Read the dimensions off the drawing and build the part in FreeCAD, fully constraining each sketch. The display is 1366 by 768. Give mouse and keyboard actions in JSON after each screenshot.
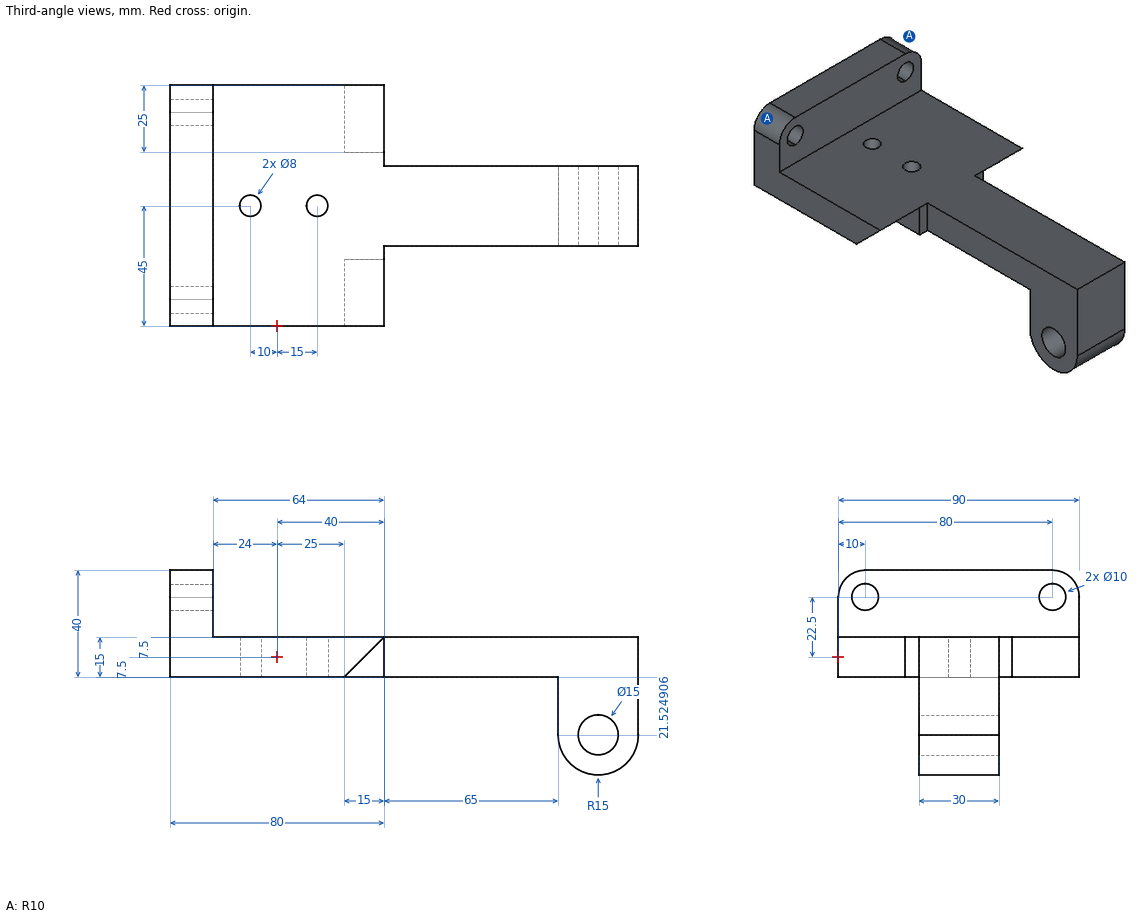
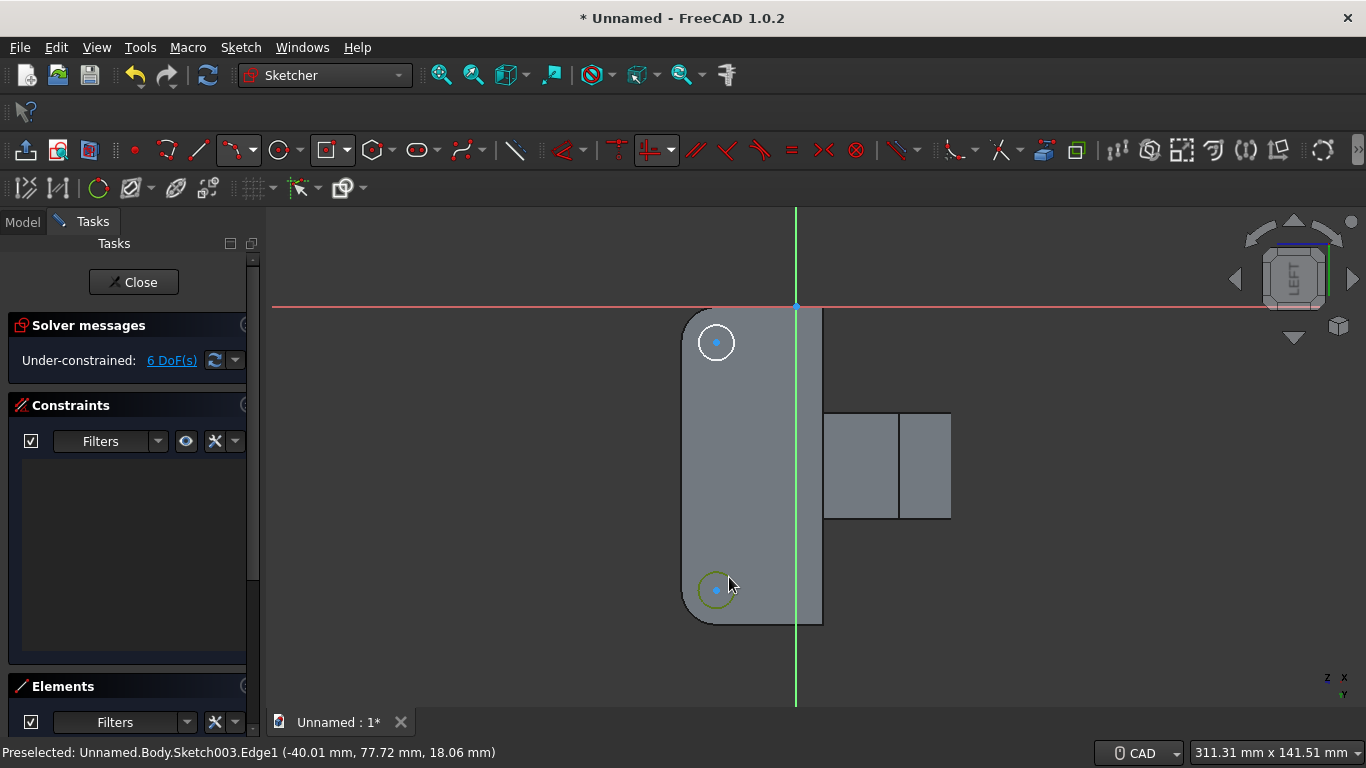
{"action": "left_click", "coordinate": [729, 330]}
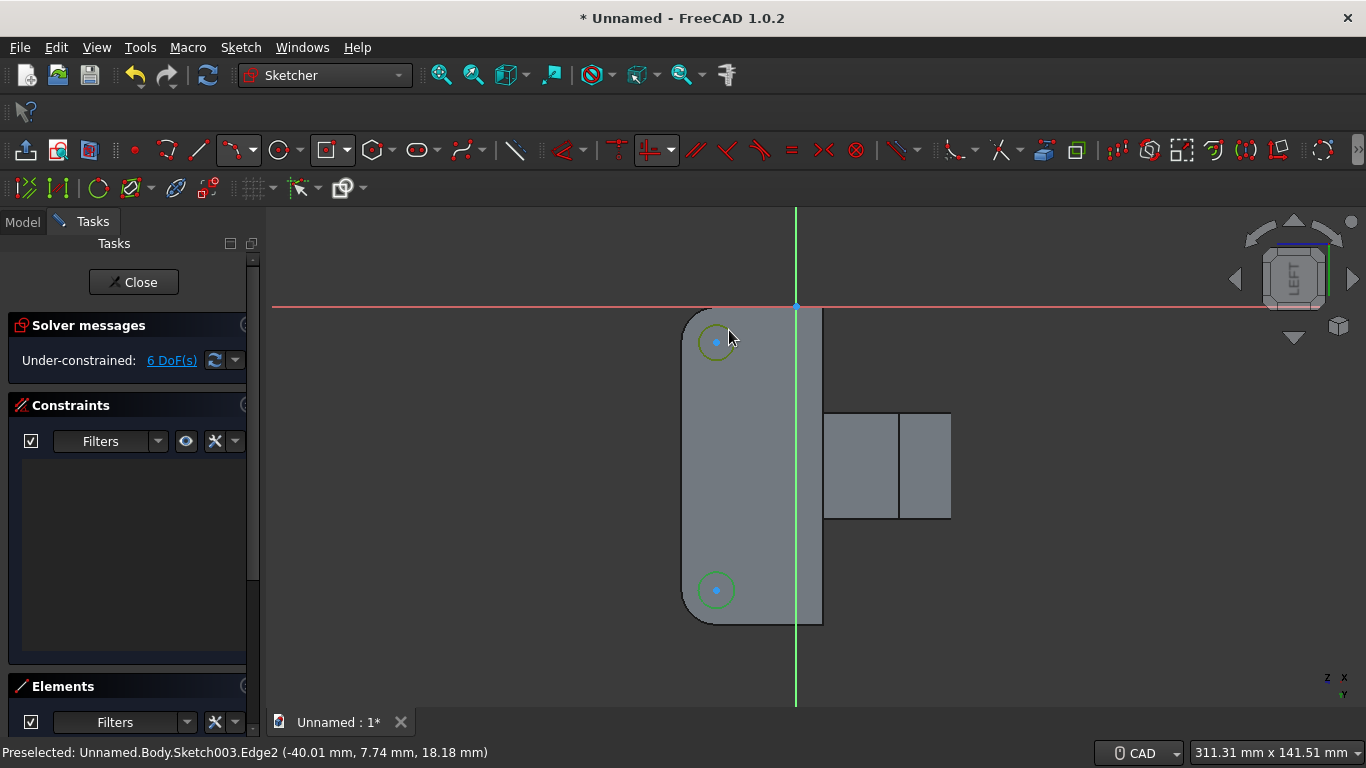
{"action": "left_click", "coordinate": [792, 150]}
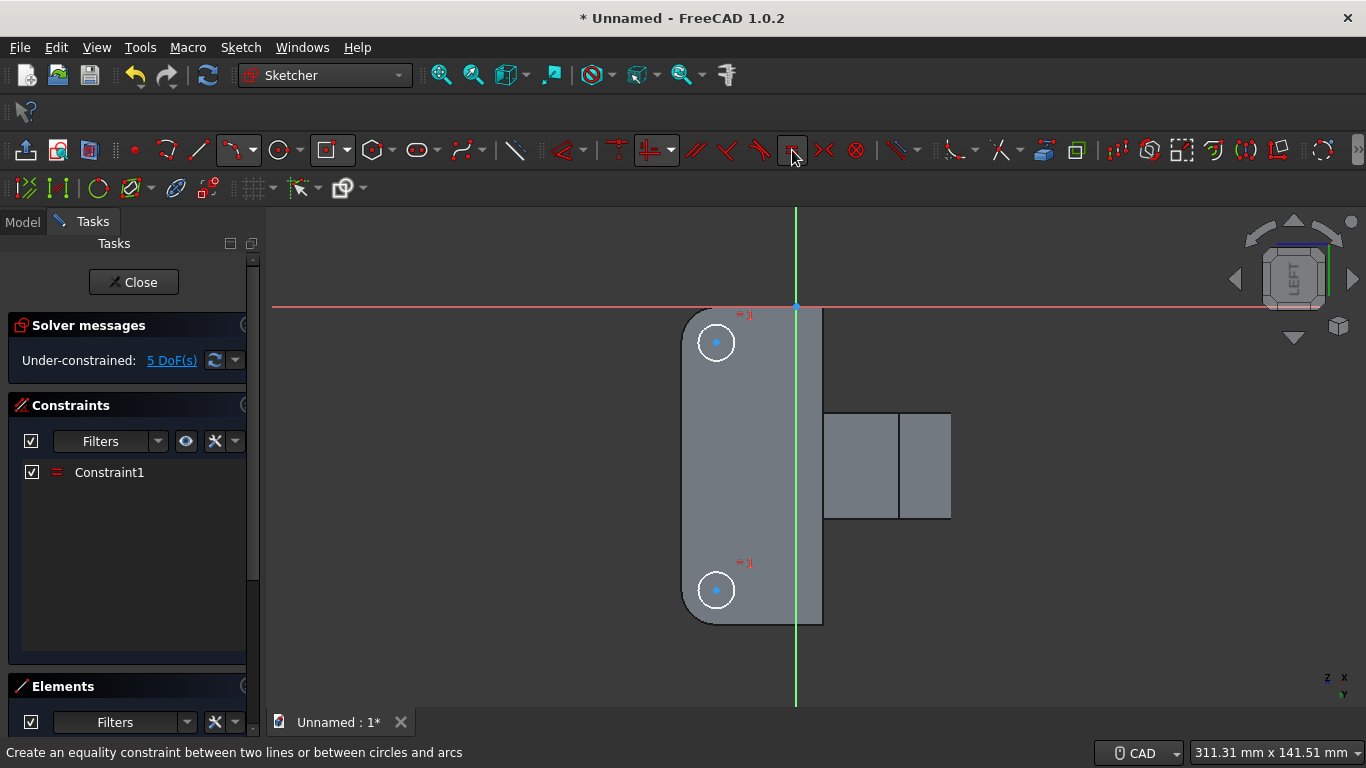
{"action": "left_click", "coordinate": [716, 590]}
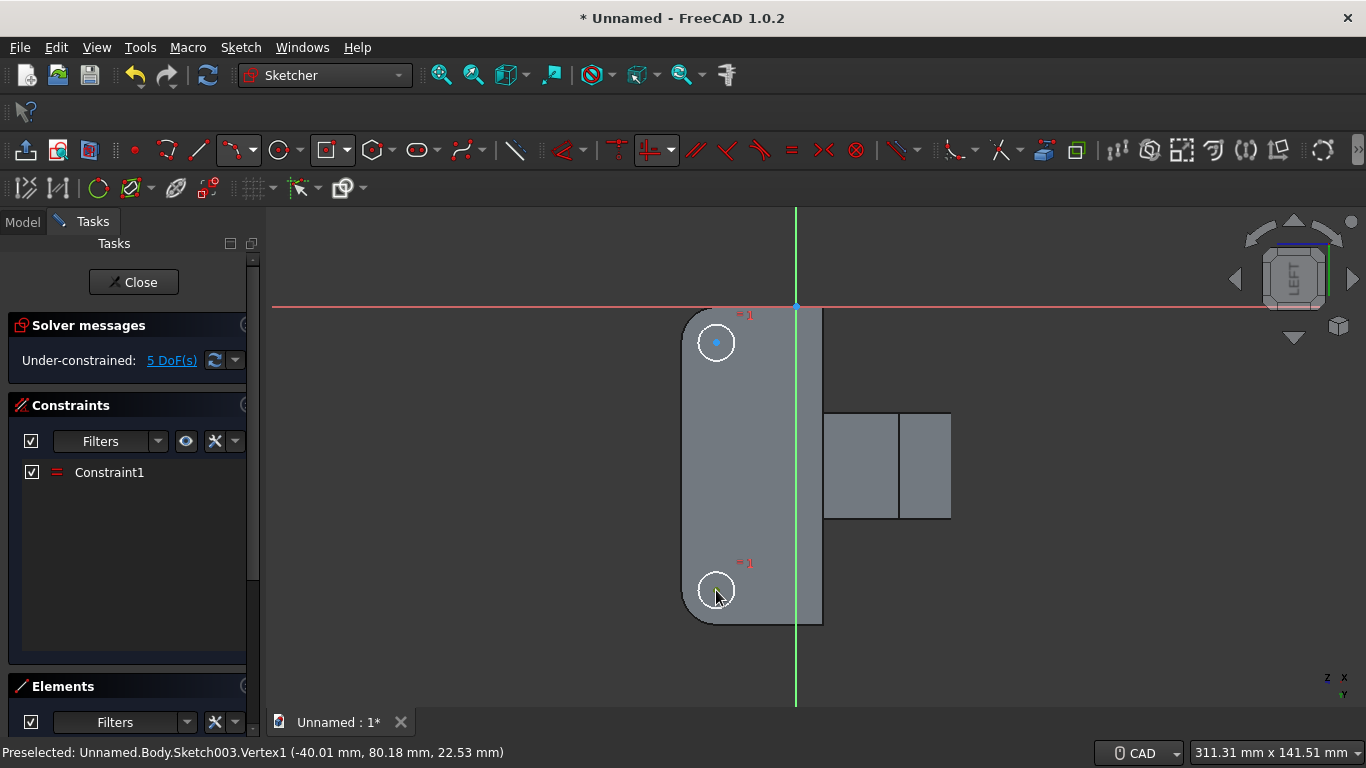
{"action": "left_click", "coordinate": [716, 343]}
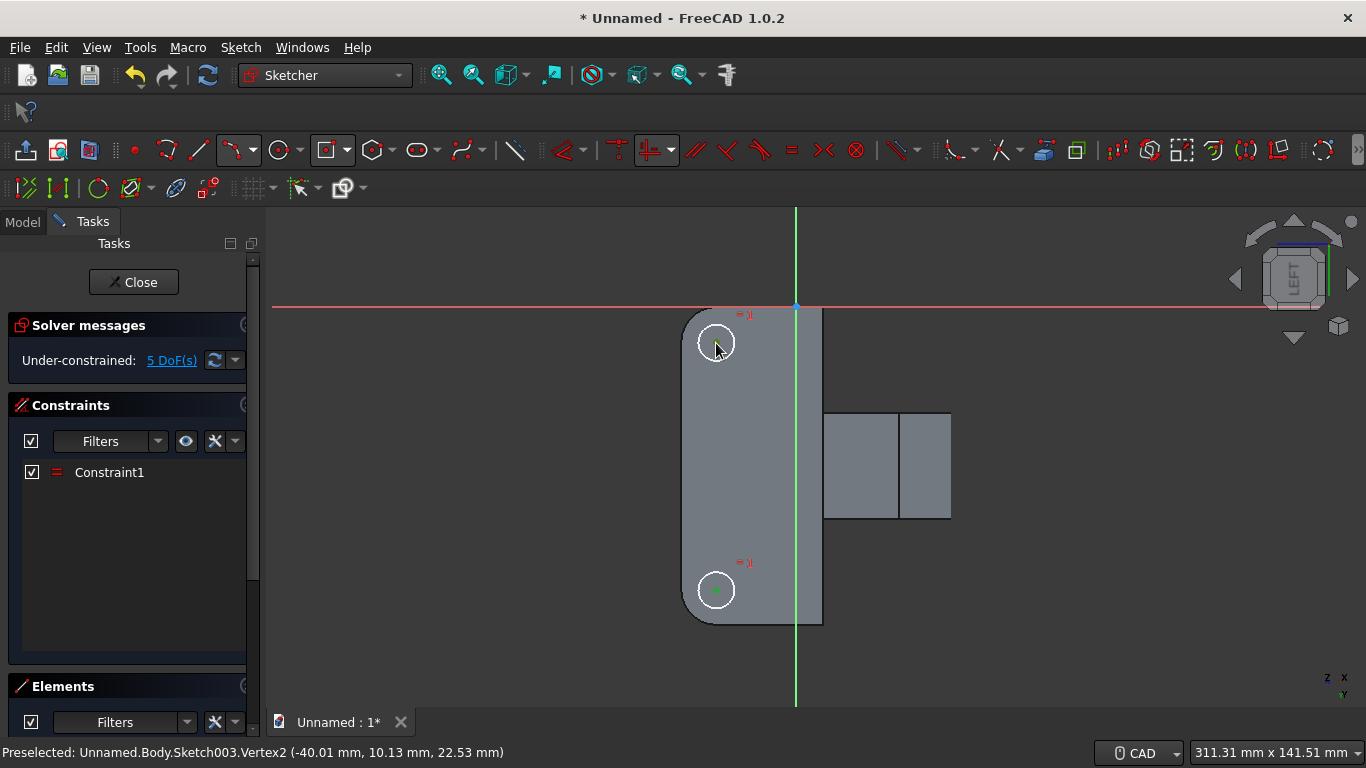
{"action": "left_click", "coordinate": [674, 150]}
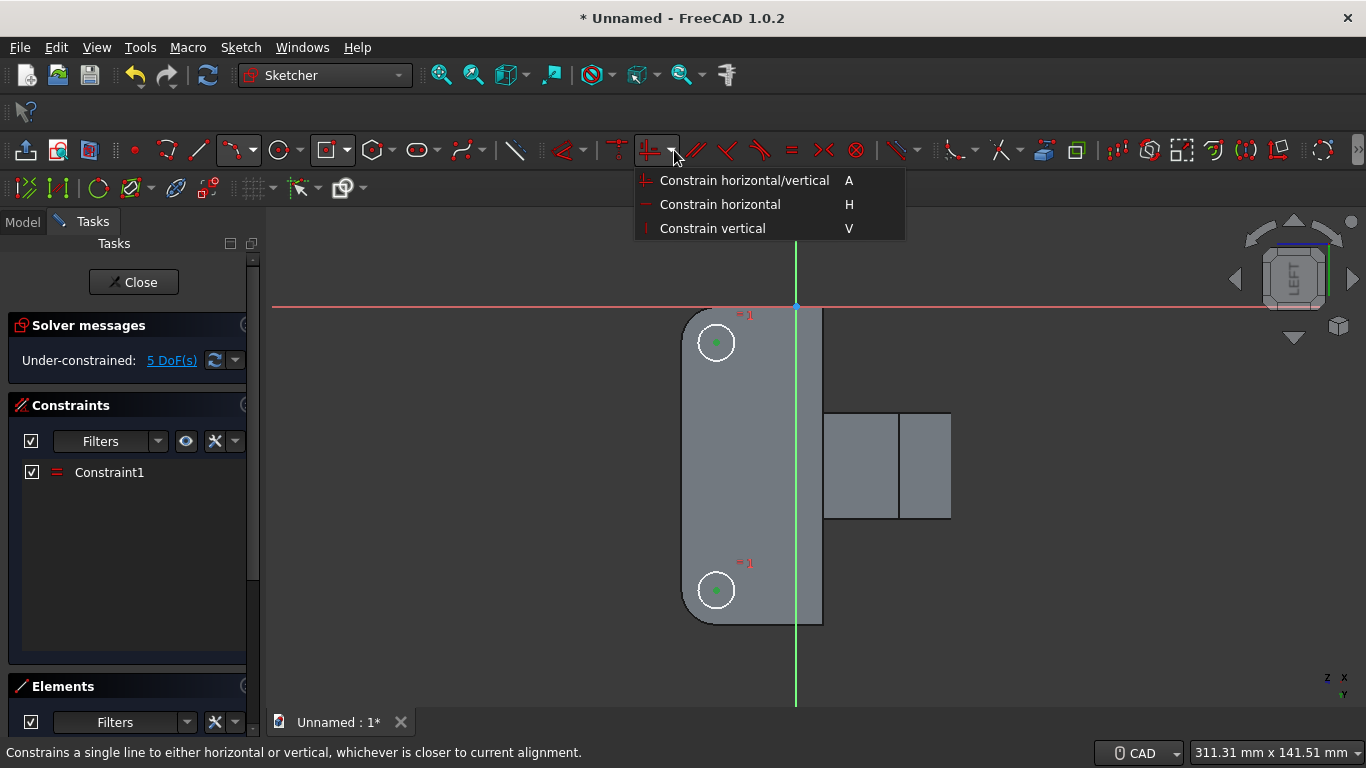
{"action": "left_click", "coordinate": [770, 228]}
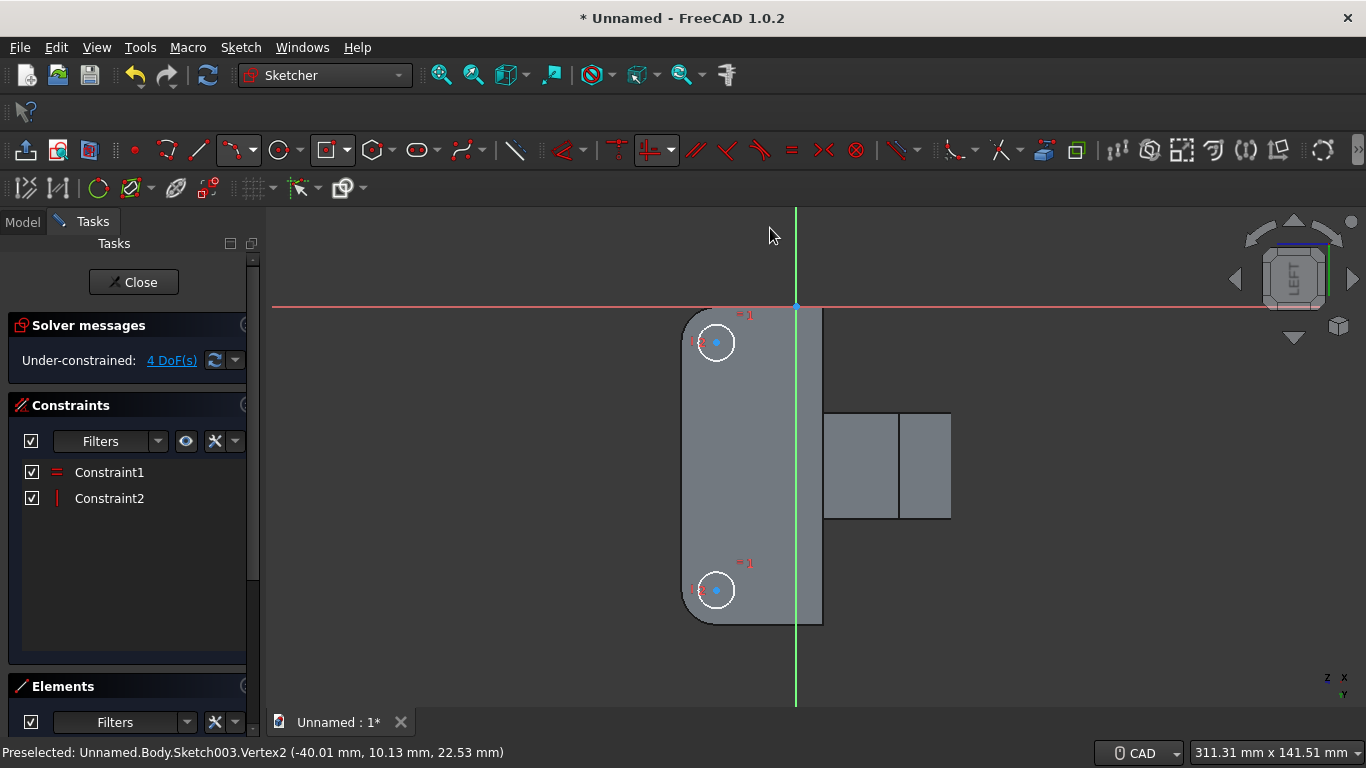
{"action": "left_click", "coordinate": [562, 150]}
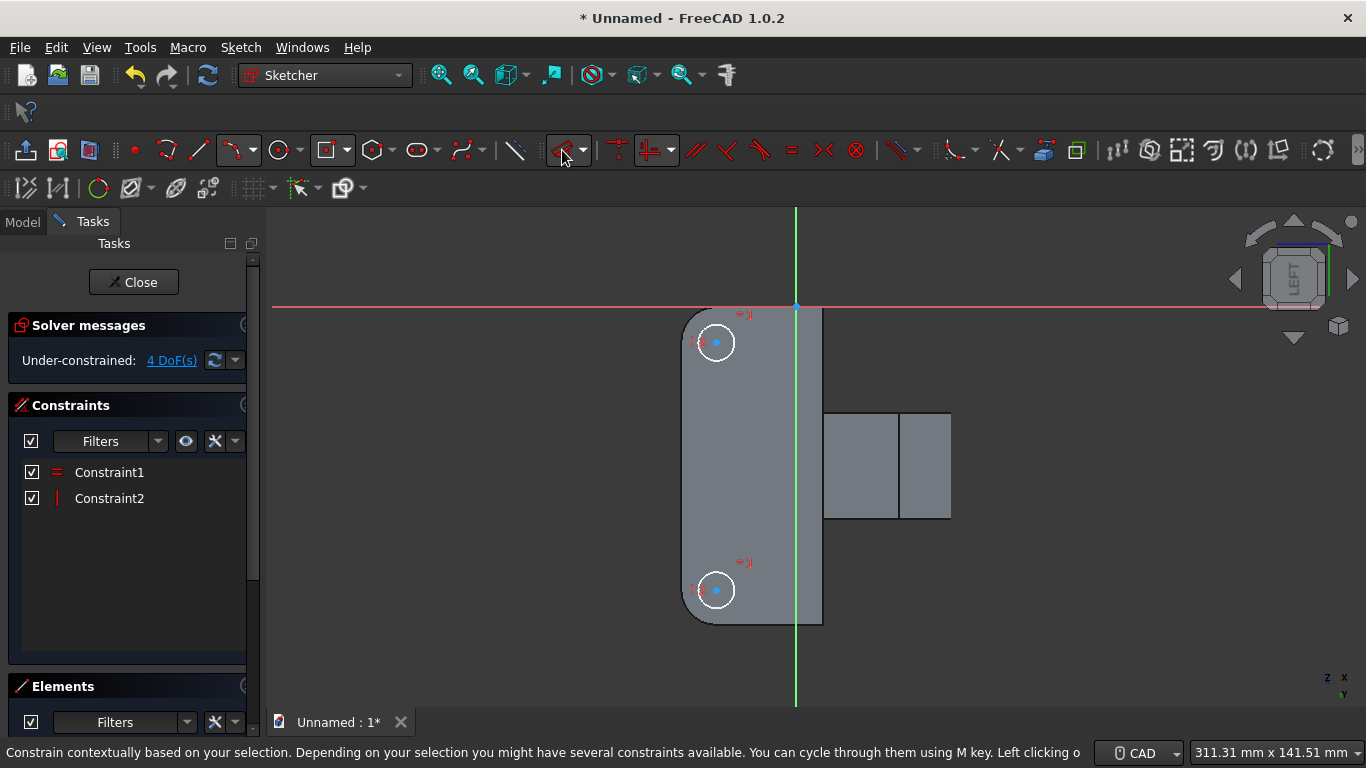
{"action": "left_click", "coordinate": [729, 577]}
{"action": "left_click", "coordinate": [751, 554]}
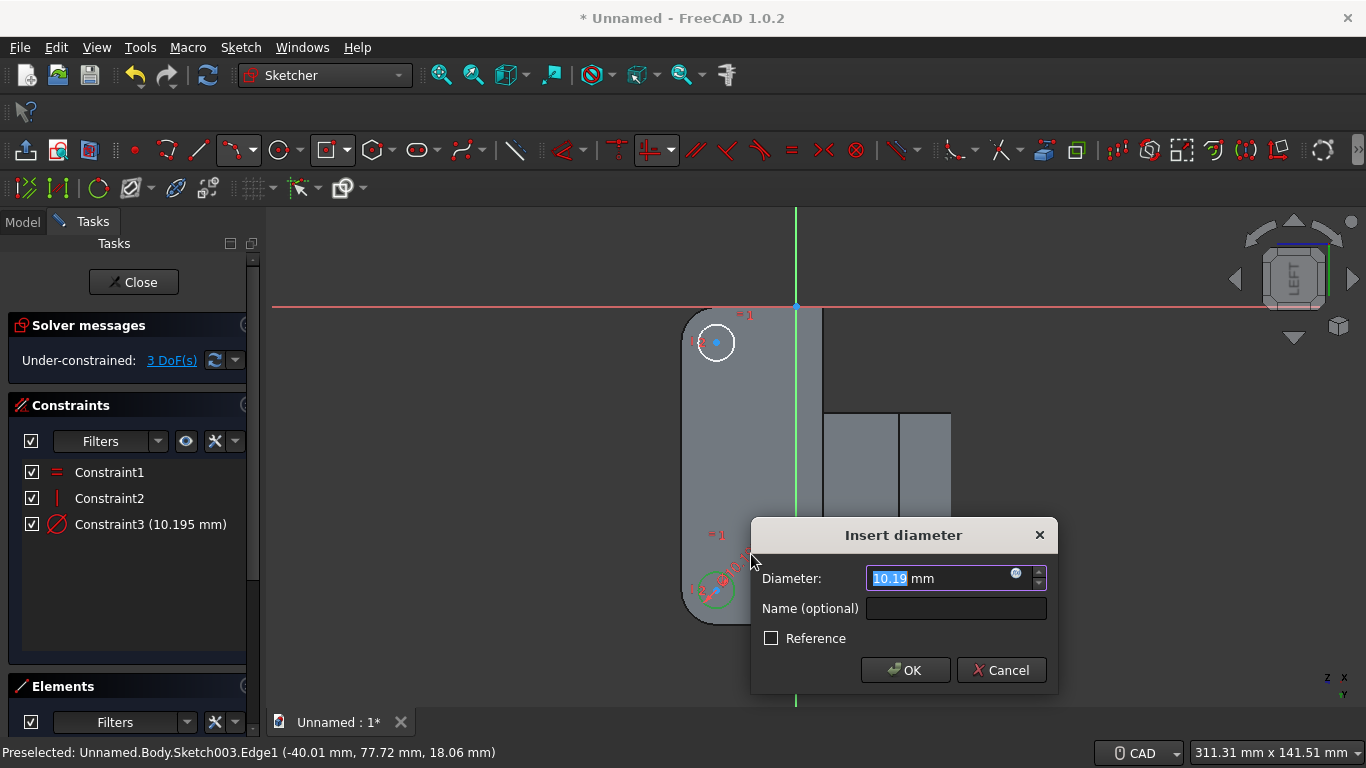
{"action": "type", "text": "10"}
{"action": "key", "text": "Return"}